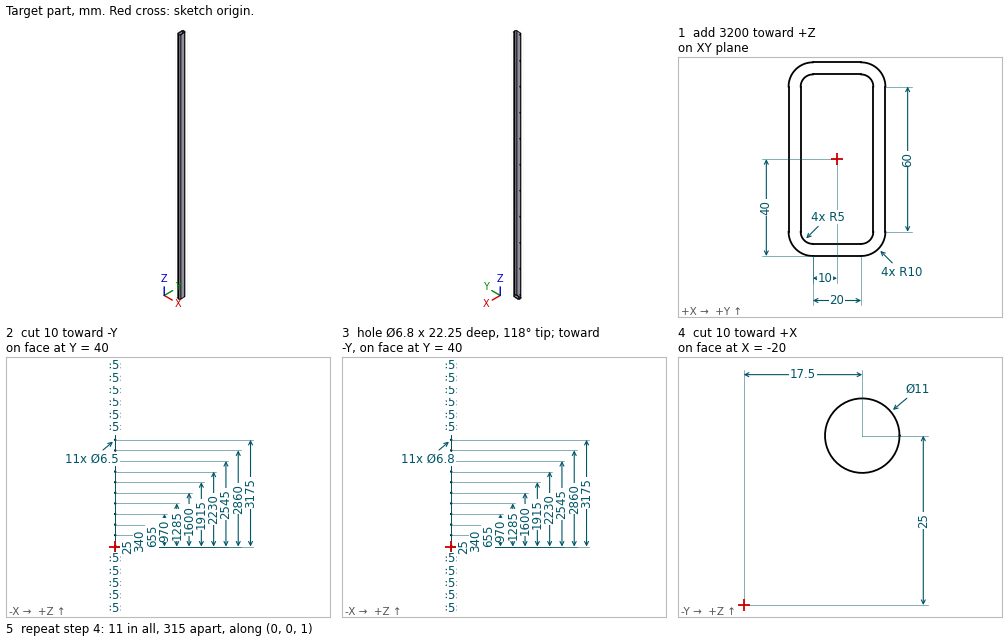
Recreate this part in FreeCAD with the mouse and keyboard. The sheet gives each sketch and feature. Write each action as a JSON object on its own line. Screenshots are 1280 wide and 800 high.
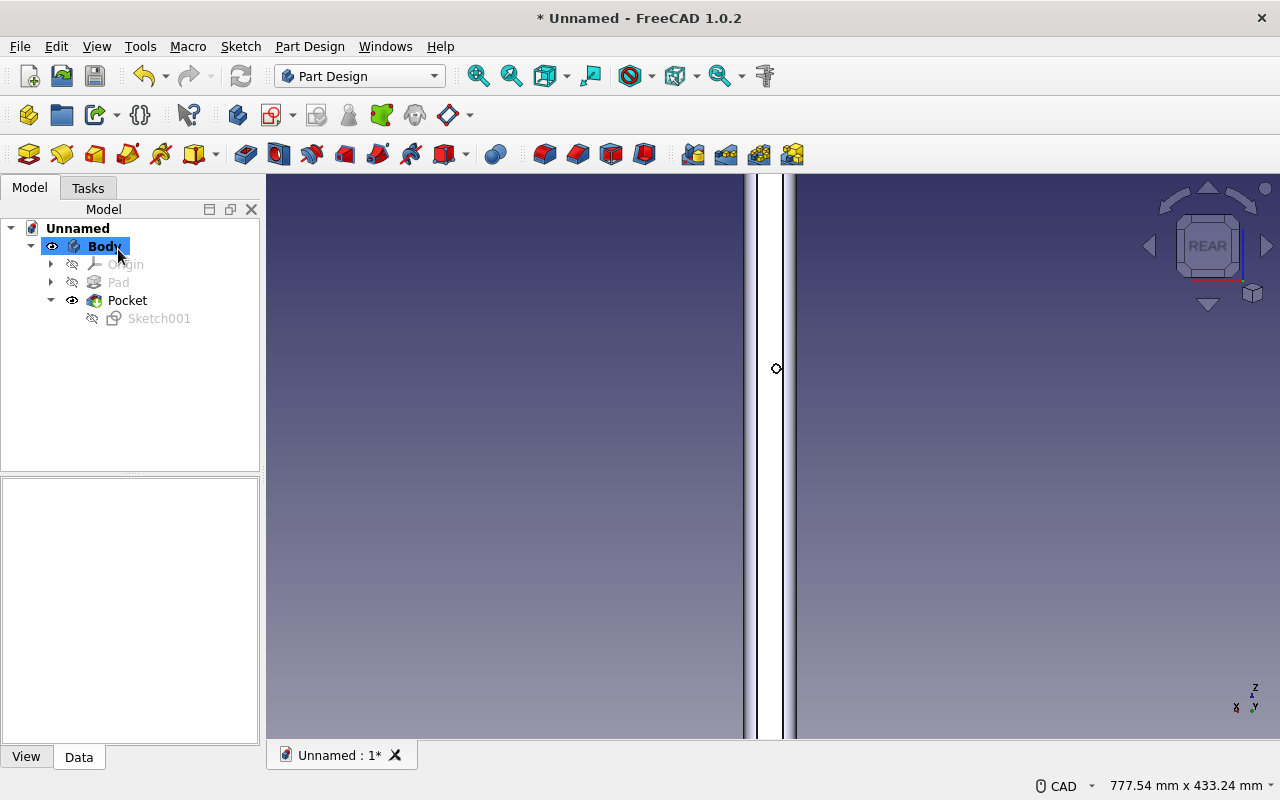
{"action": "key", "text": "v f"}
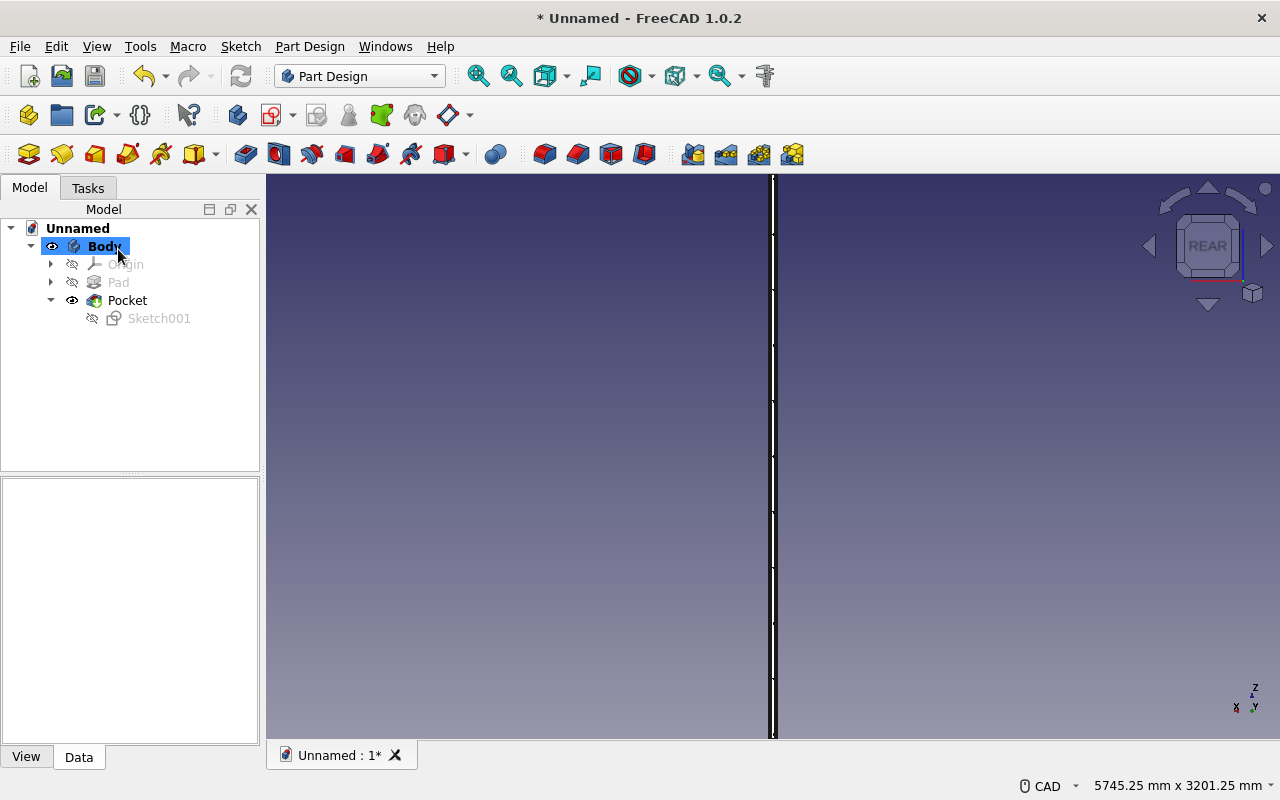
{"action": "scroll", "coordinate": [773, 213], "scroll_direction": "up", "scroll_amount": 10}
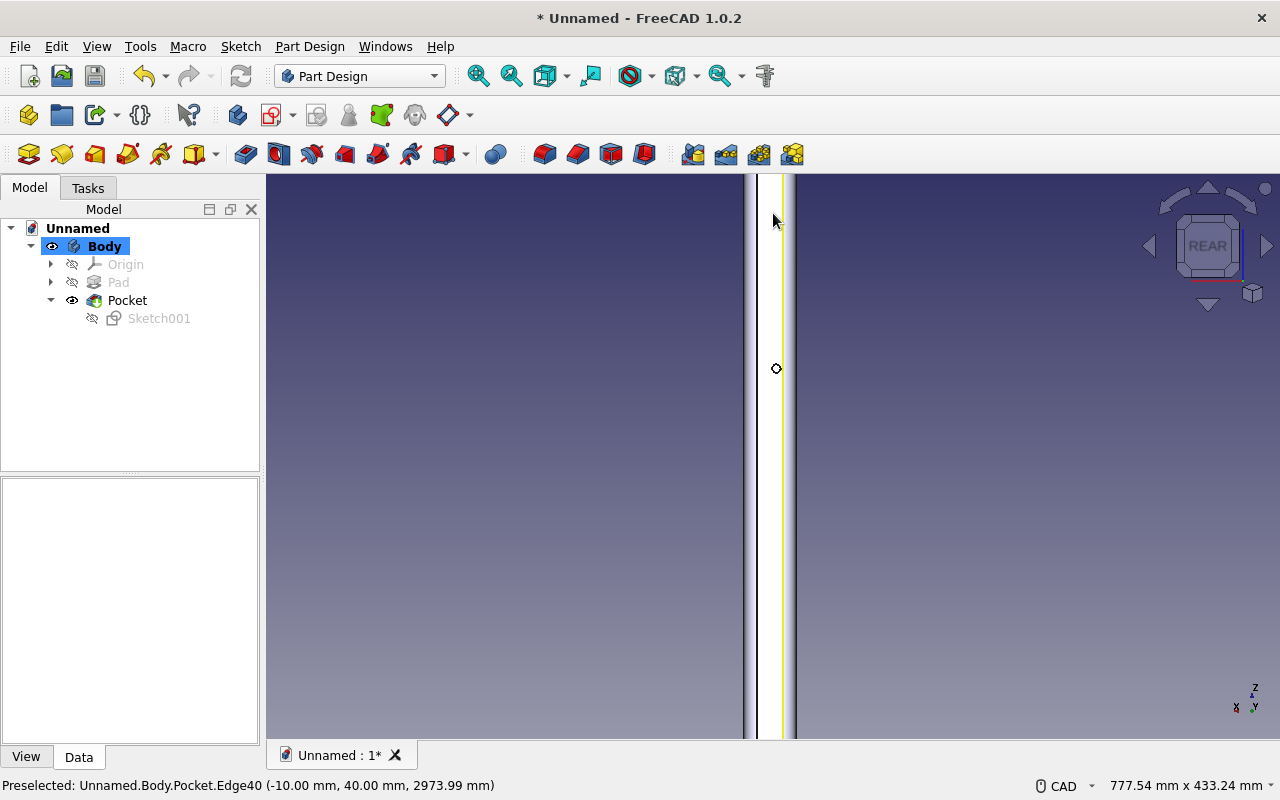
{"action": "left_click", "coordinate": [770, 222]}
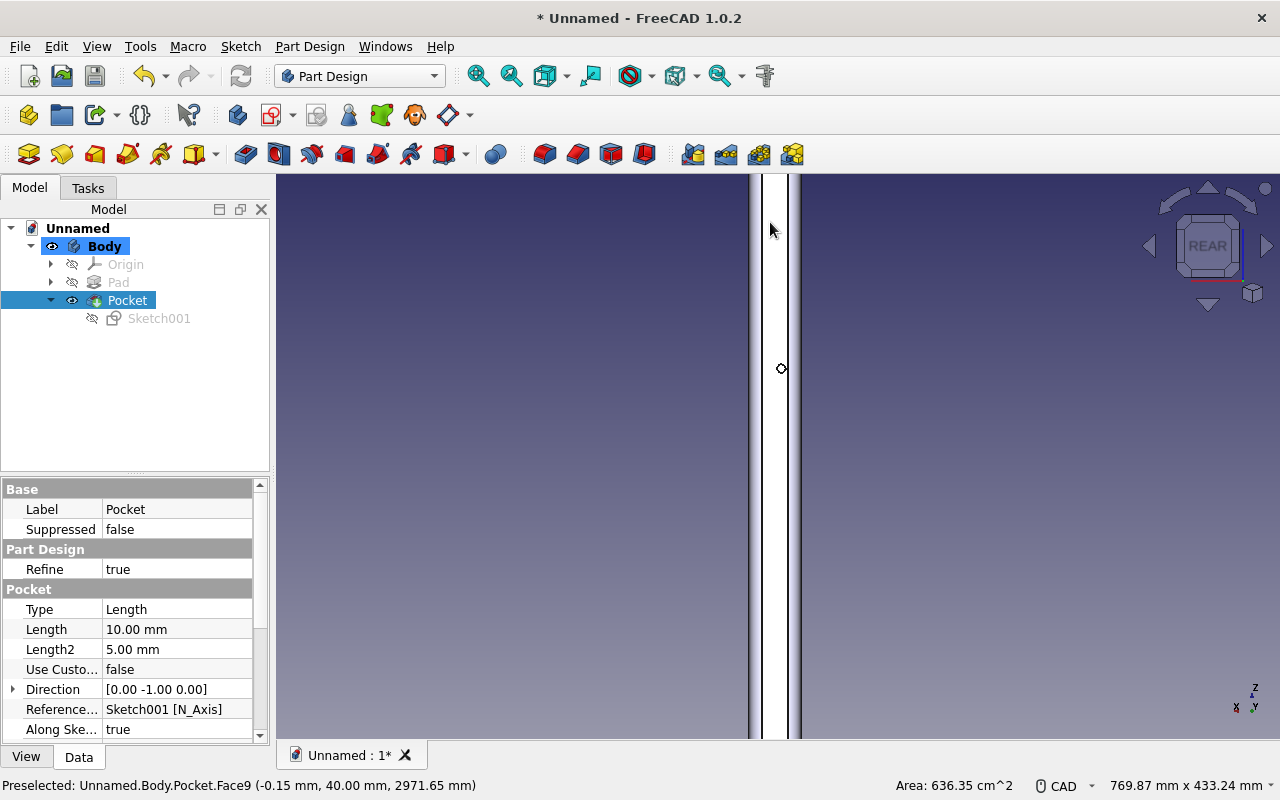
{"action": "left_click", "coordinate": [270, 116]}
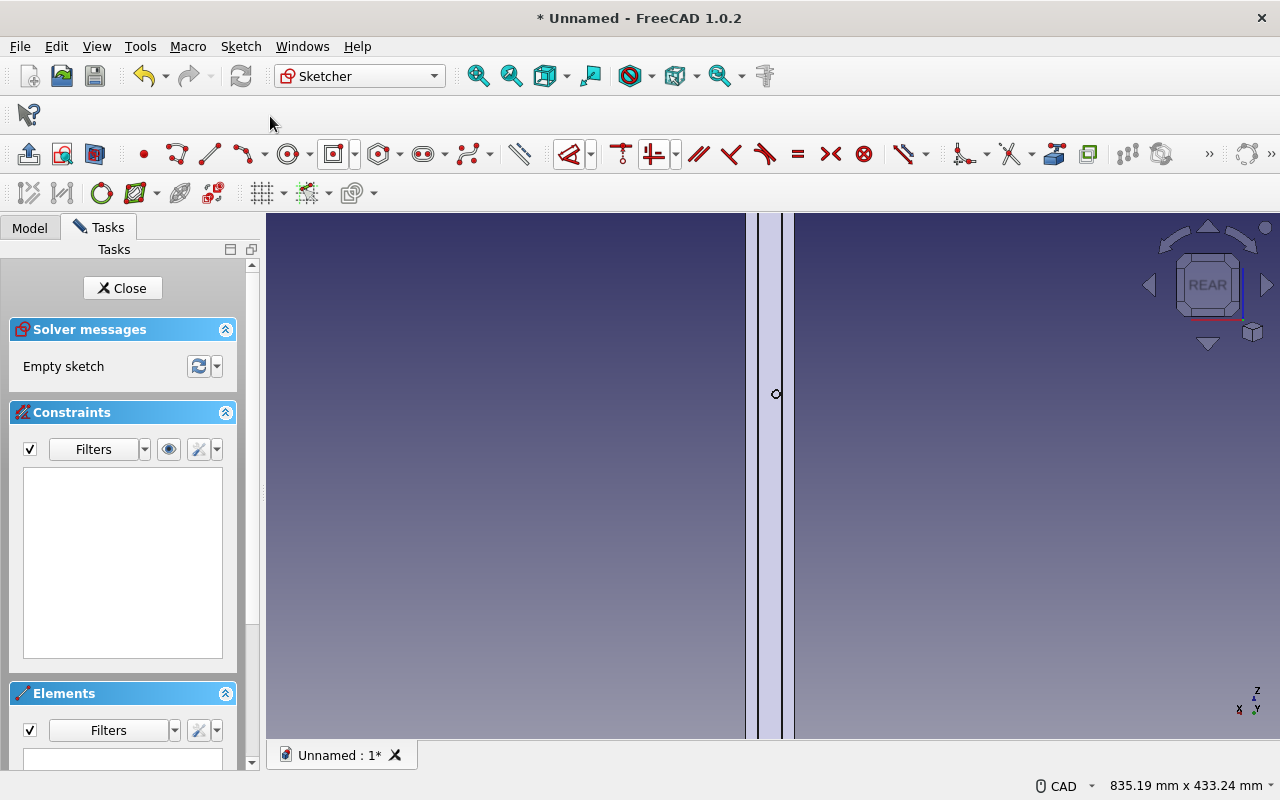
{"action": "scroll", "coordinate": [697, 330], "scroll_direction": "down", "scroll_amount": 12}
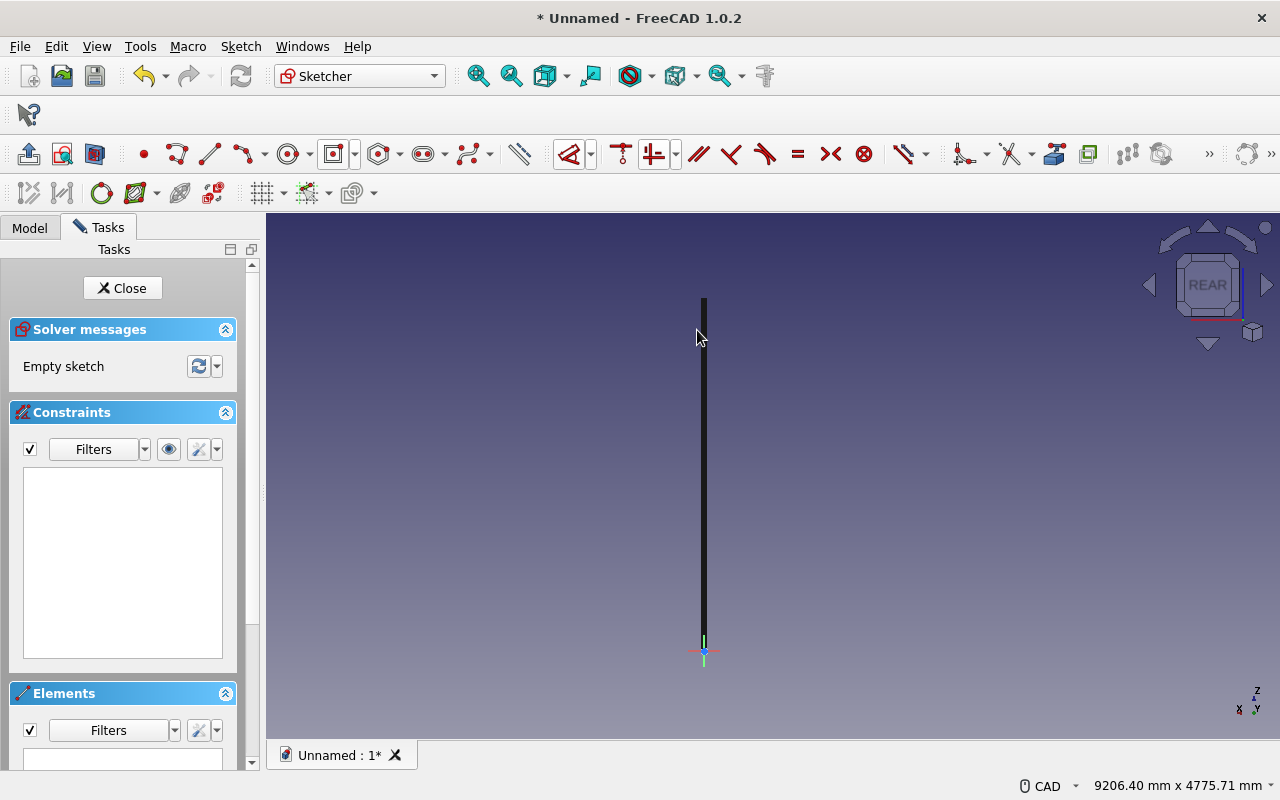
{"action": "left_click", "coordinate": [288, 154]}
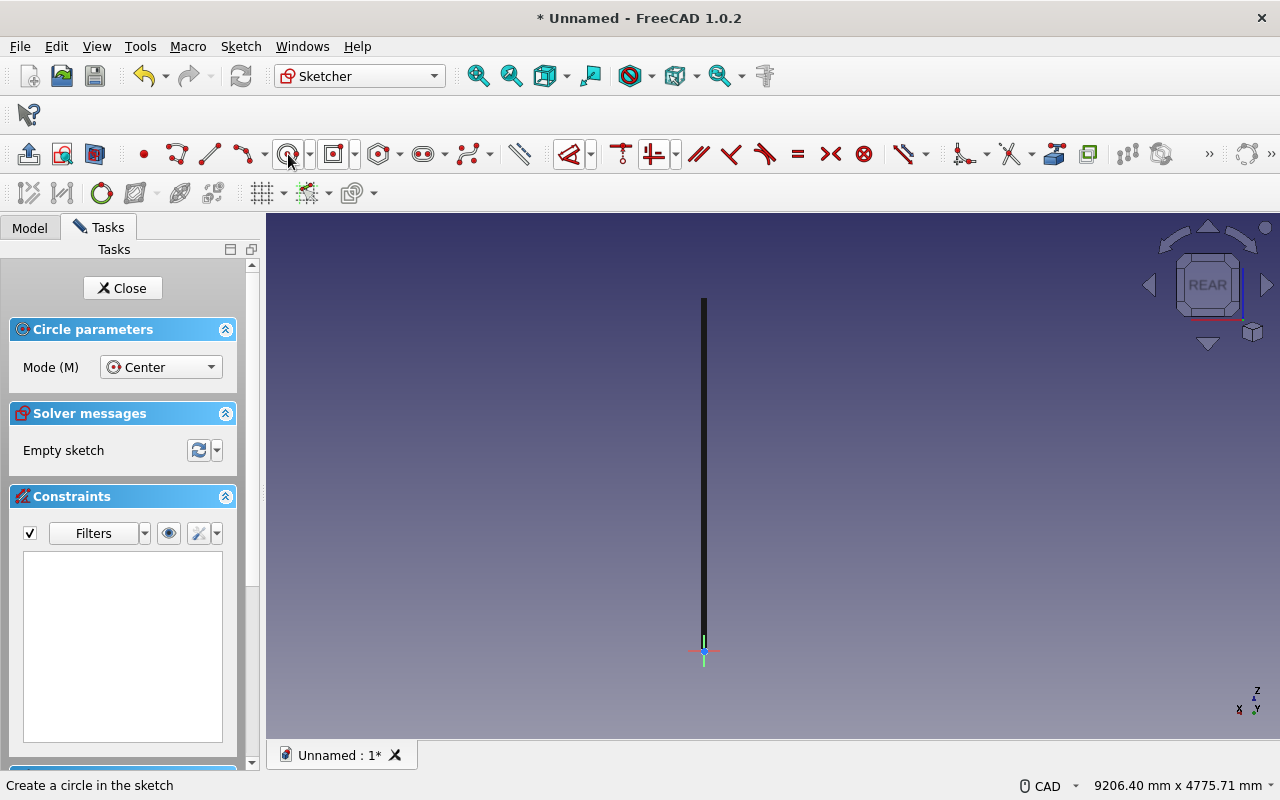
{"action": "scroll", "coordinate": [705, 301], "scroll_direction": "up", "scroll_amount": 21}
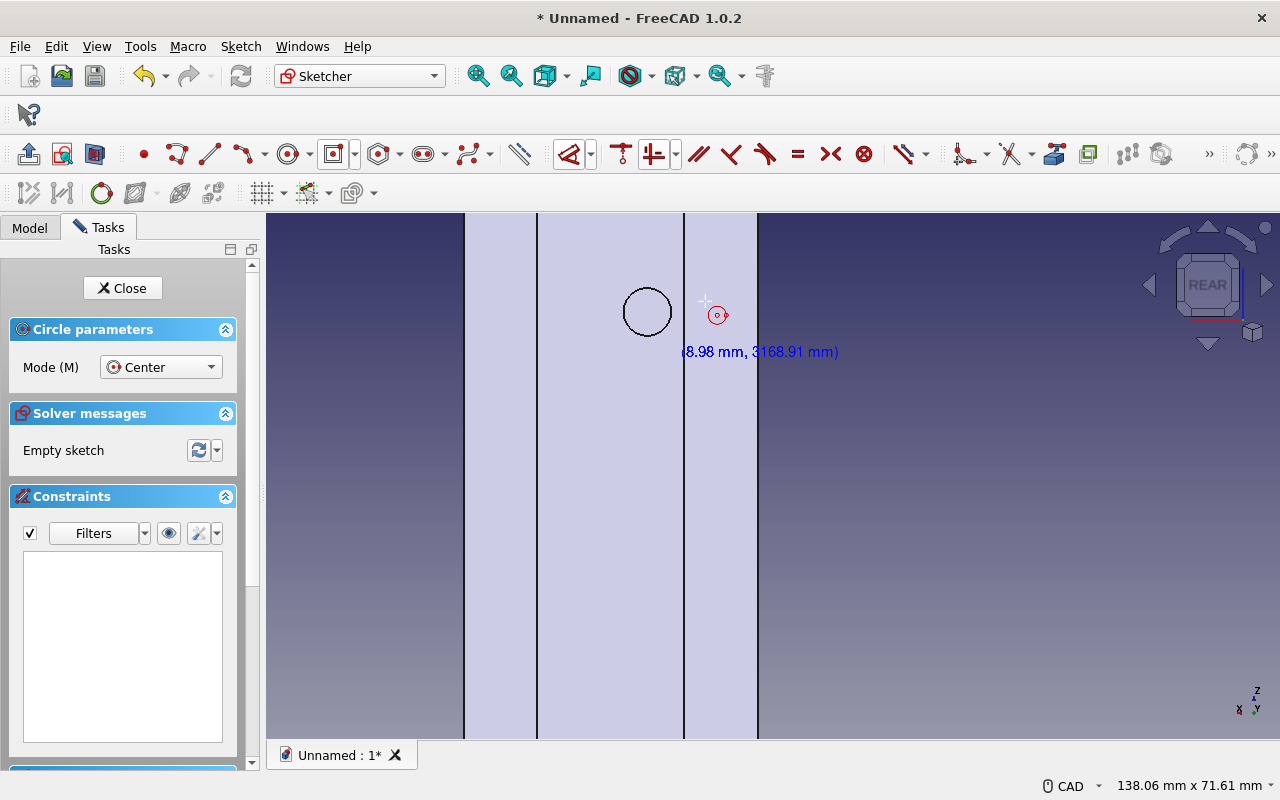
{"action": "left_click", "coordinate": [647, 312]}
{"action": "left_click", "coordinate": [665, 294]}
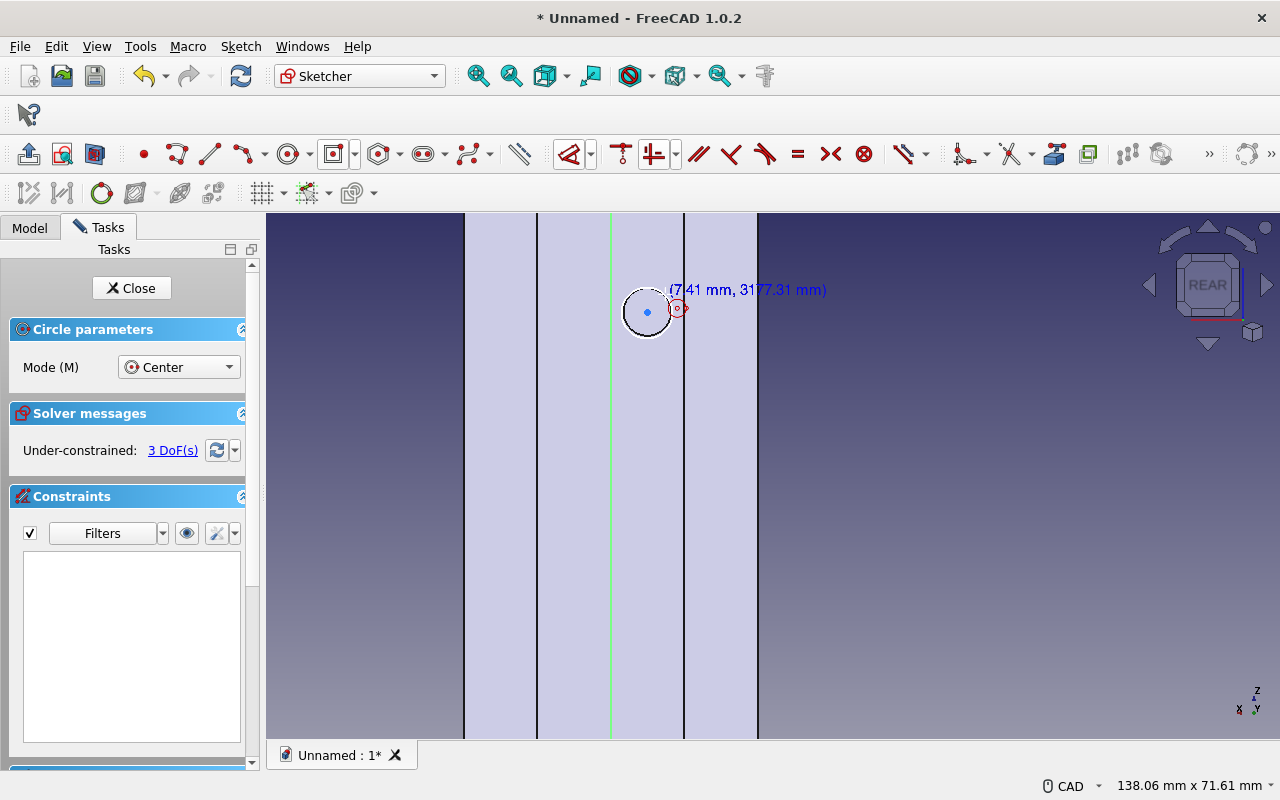
{"action": "scroll", "coordinate": [704, 476], "scroll_direction": "down", "scroll_amount": 15}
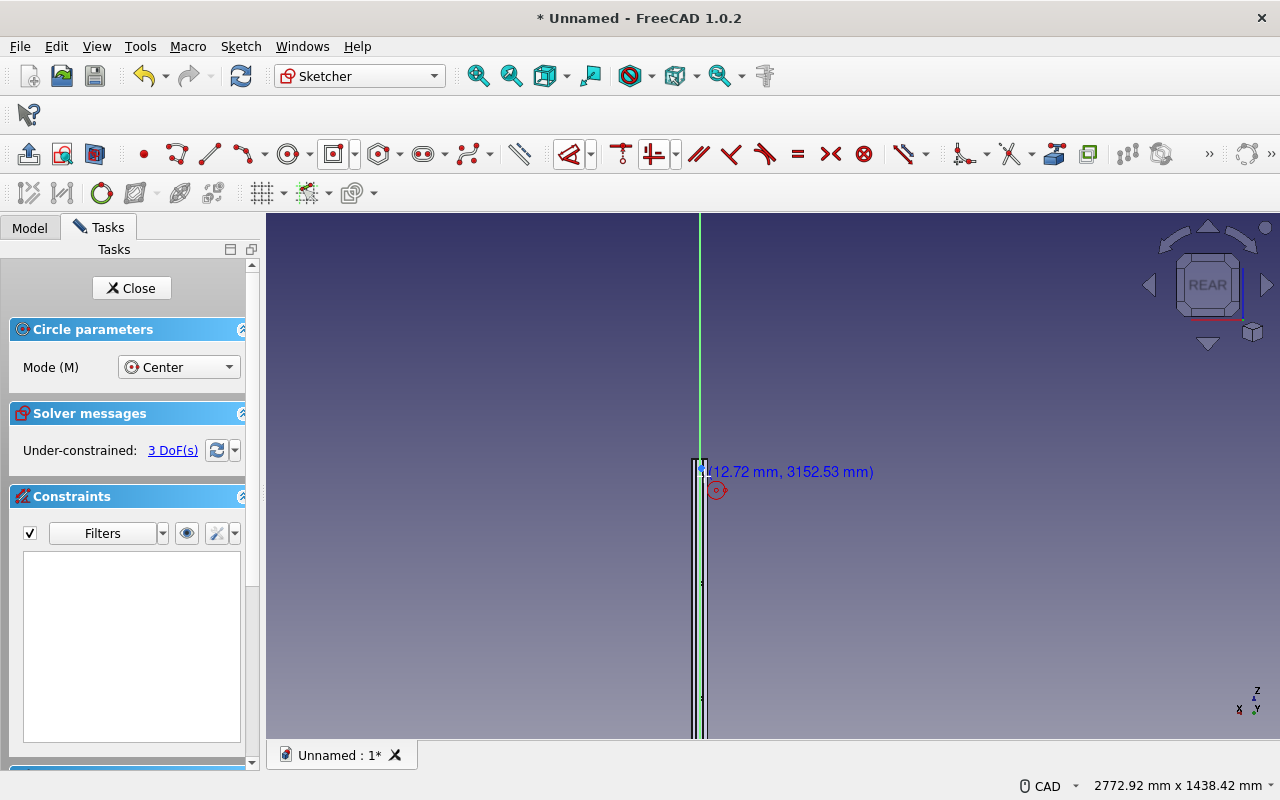
{"action": "scroll", "coordinate": [706, 241], "scroll_direction": "down", "scroll_amount": 6}